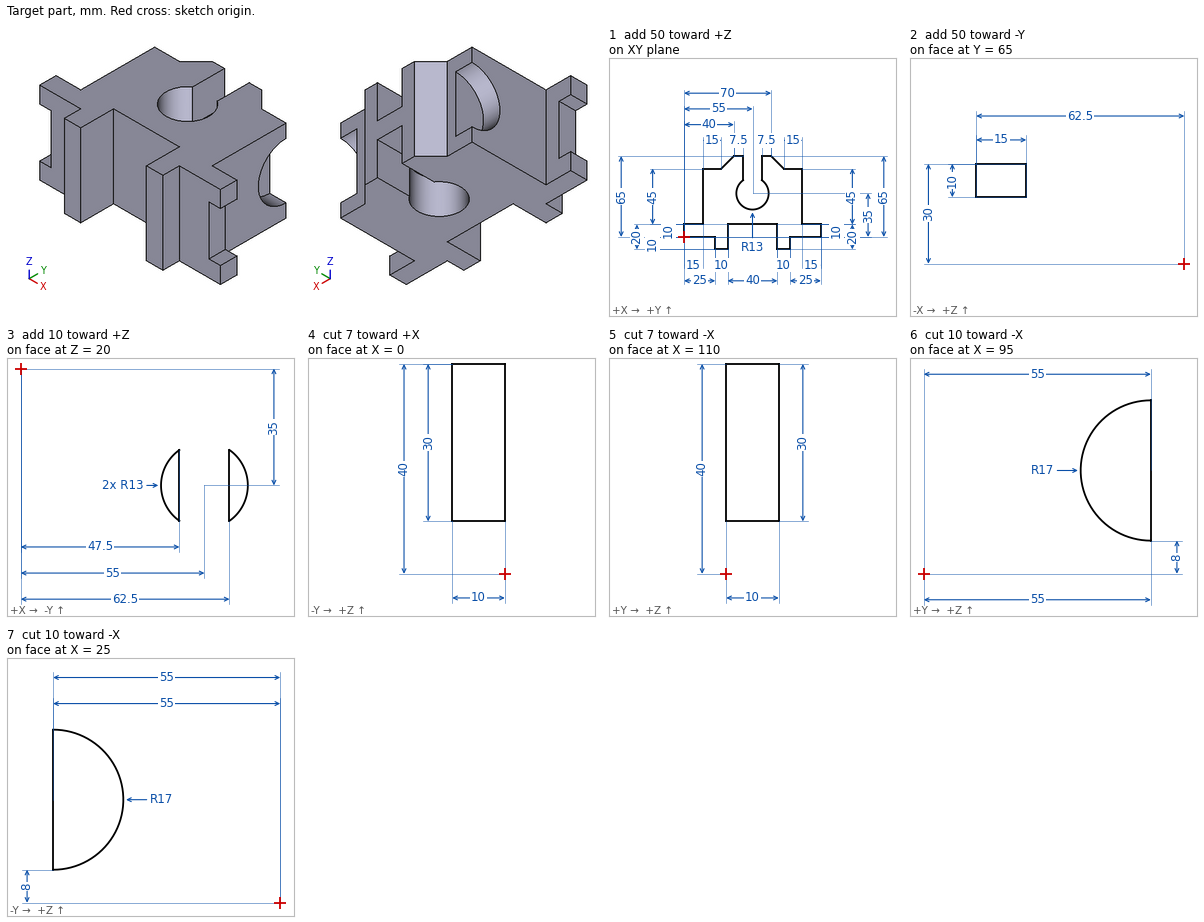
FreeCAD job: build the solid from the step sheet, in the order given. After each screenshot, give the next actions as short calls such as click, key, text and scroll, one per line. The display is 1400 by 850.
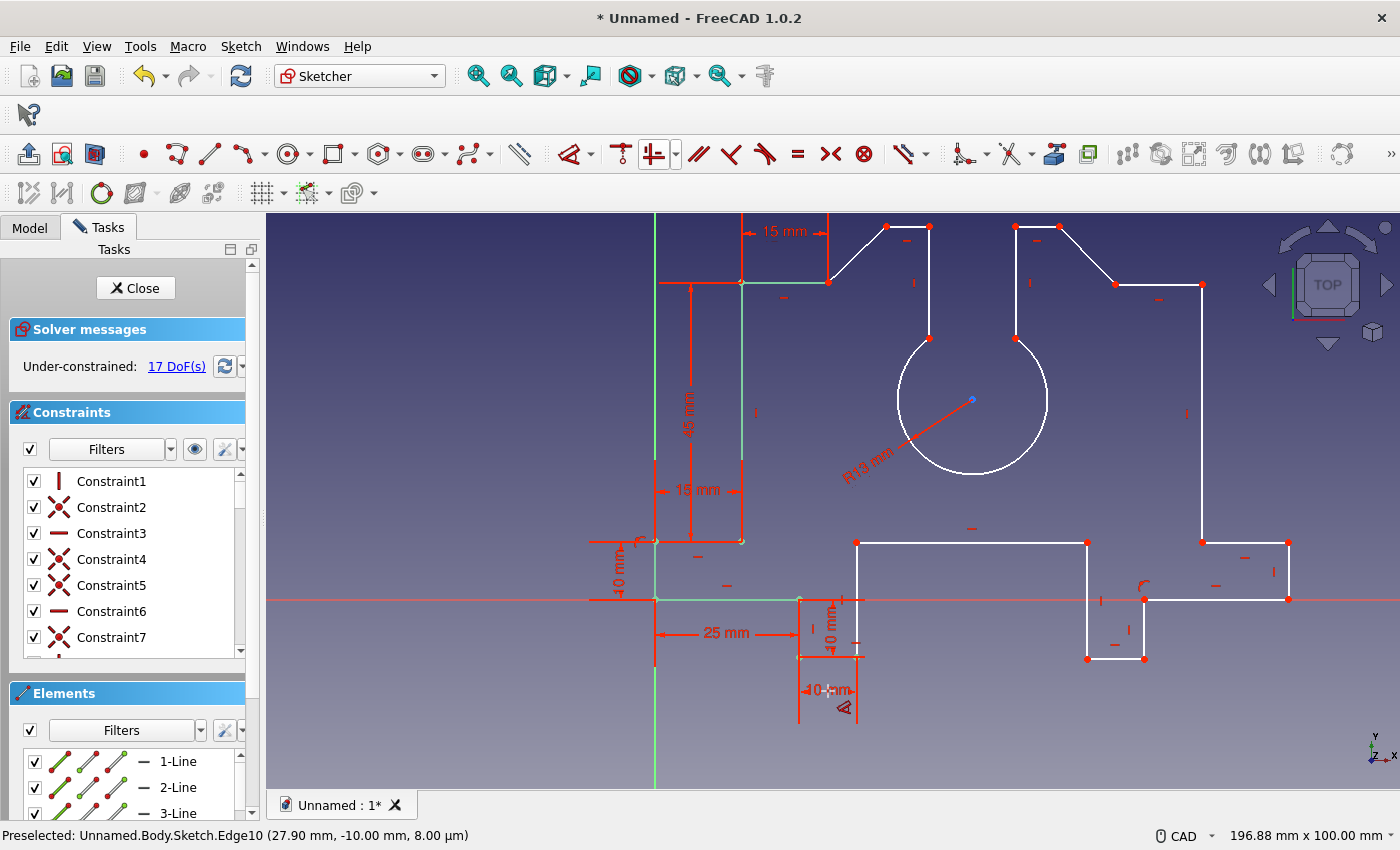
click(857, 623)
click(823, 574)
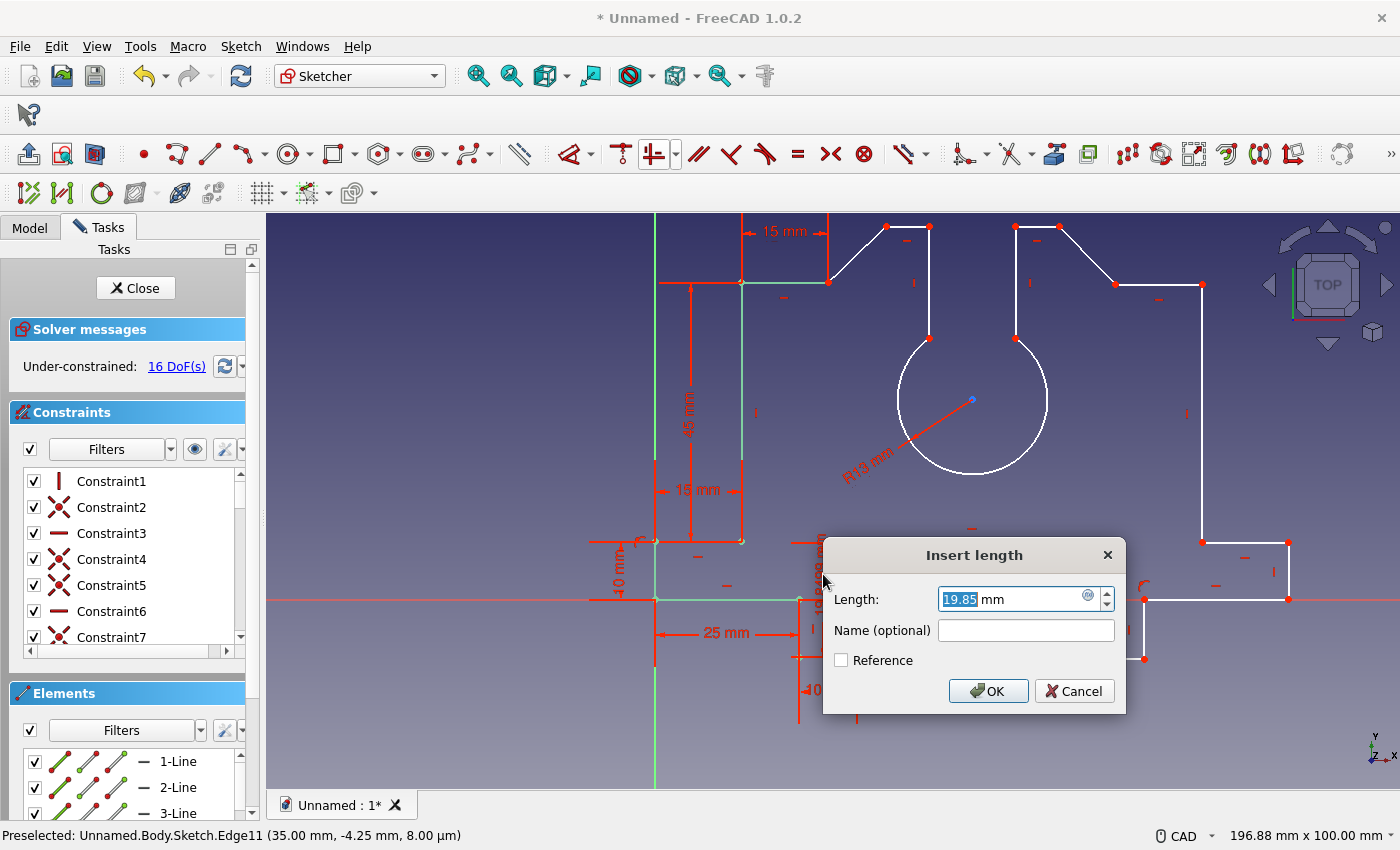
text(20)
key(Return)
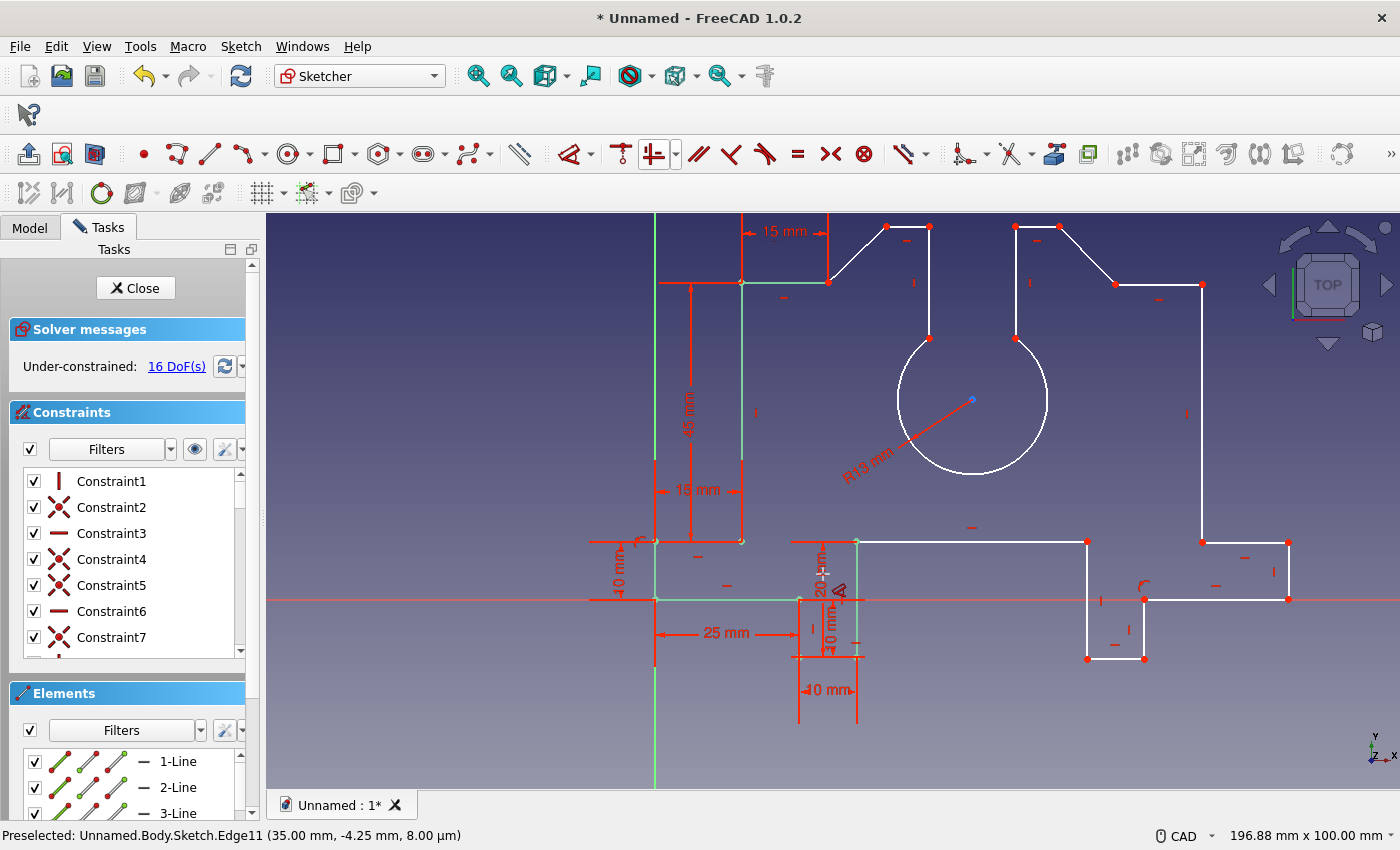
click(926, 542)
click(972, 576)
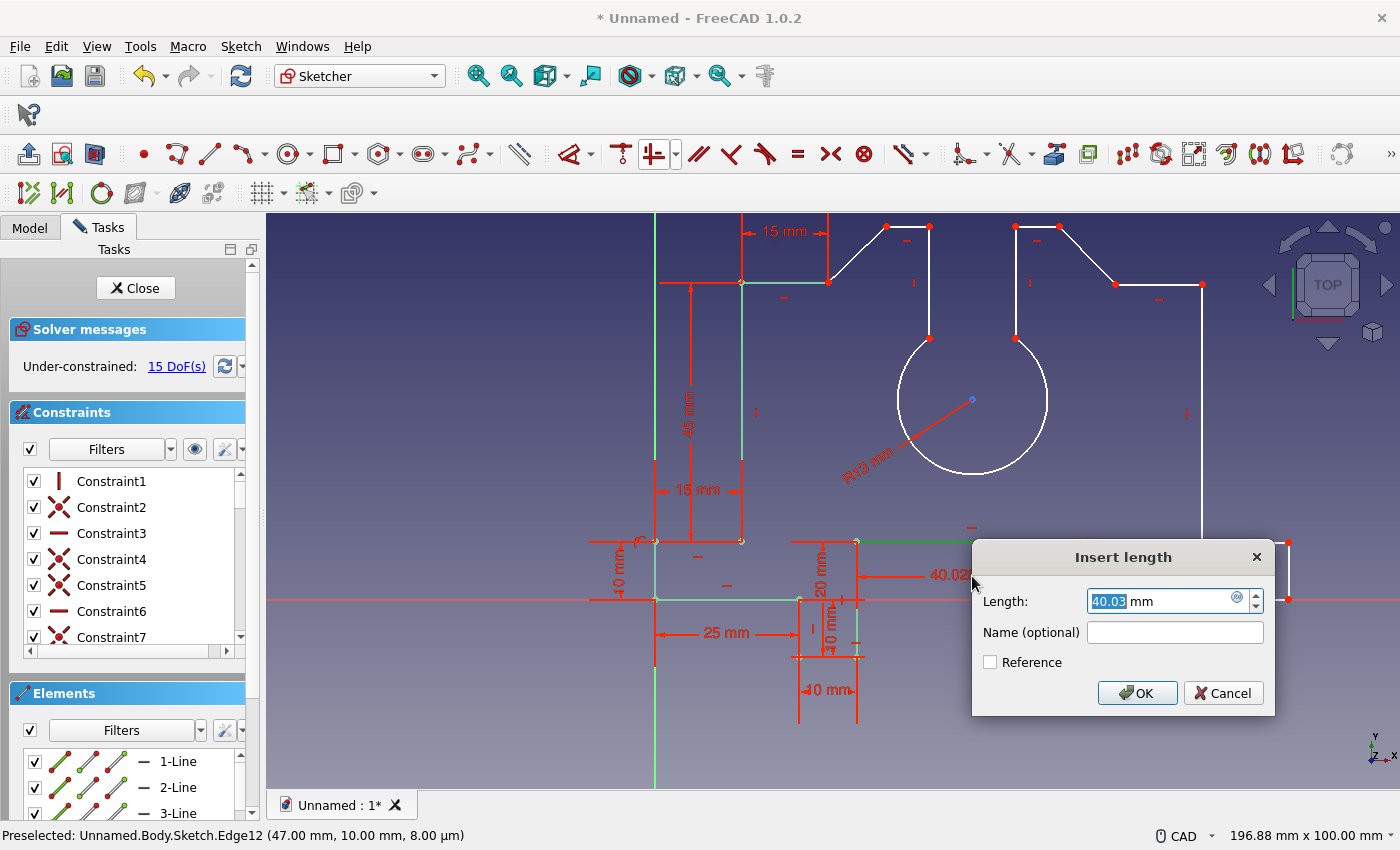
text(40)
key(Return)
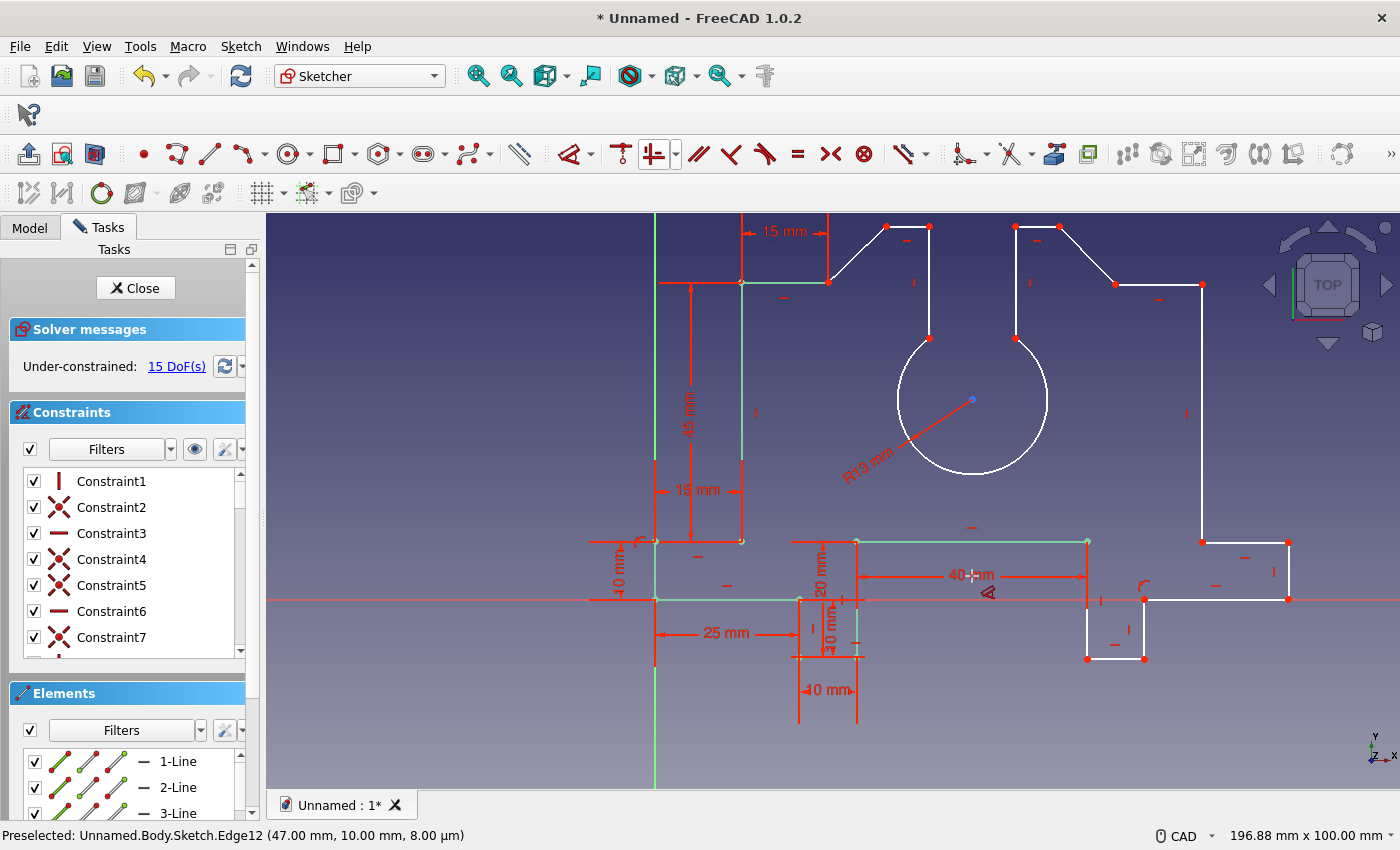
click(1087, 577)
click(1121, 574)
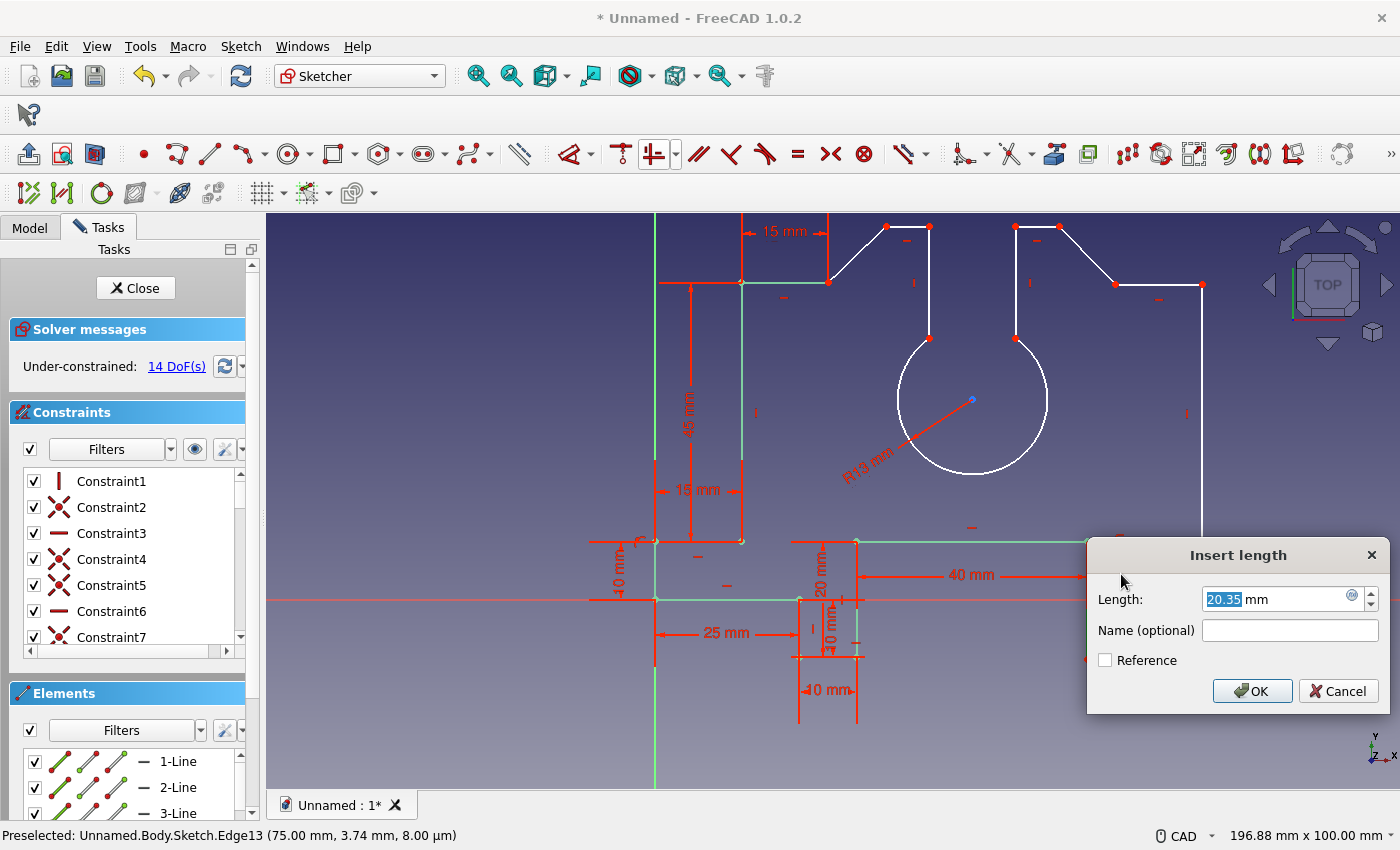
text(20)
key(Return)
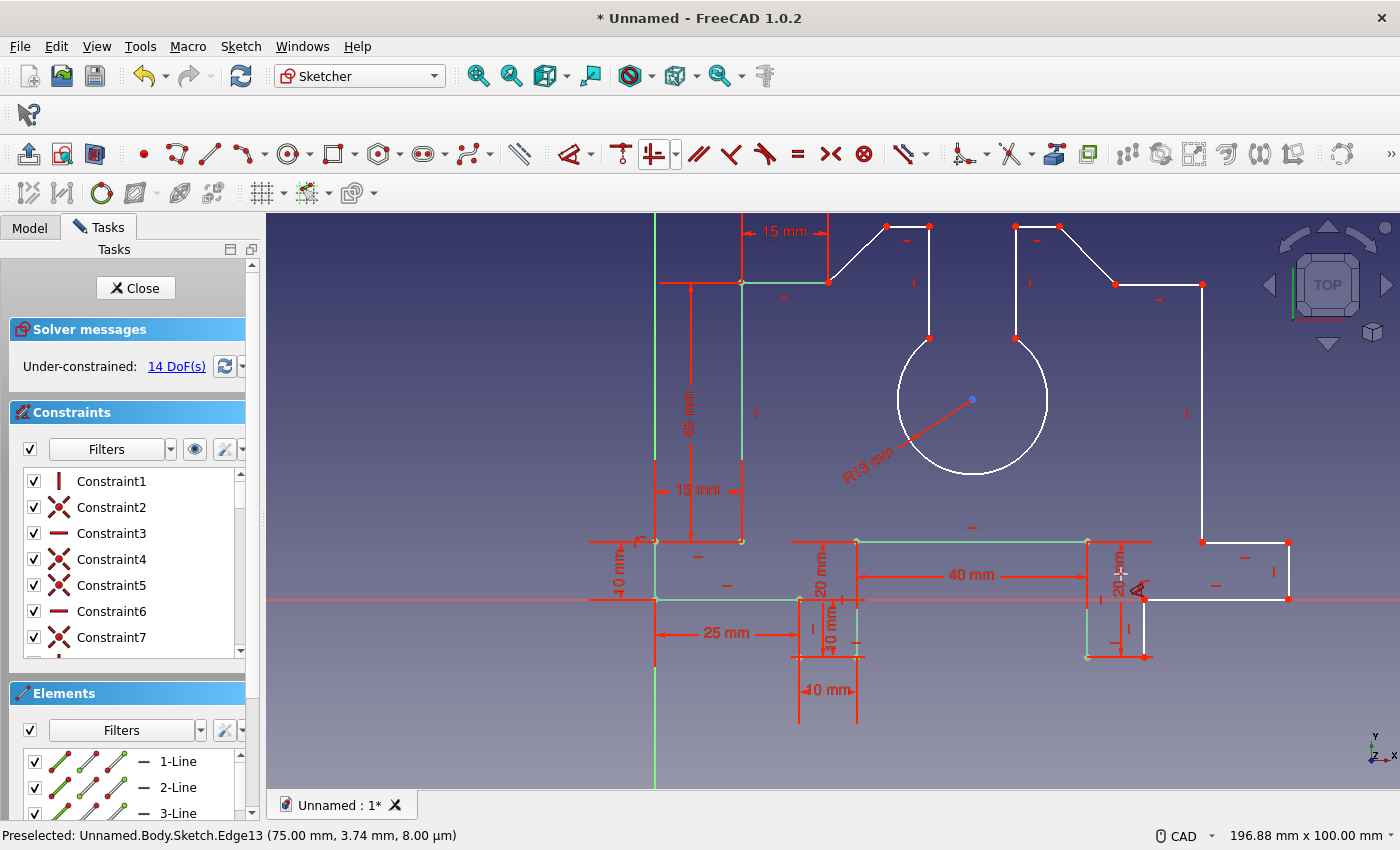
click(1104, 657)
click(1116, 691)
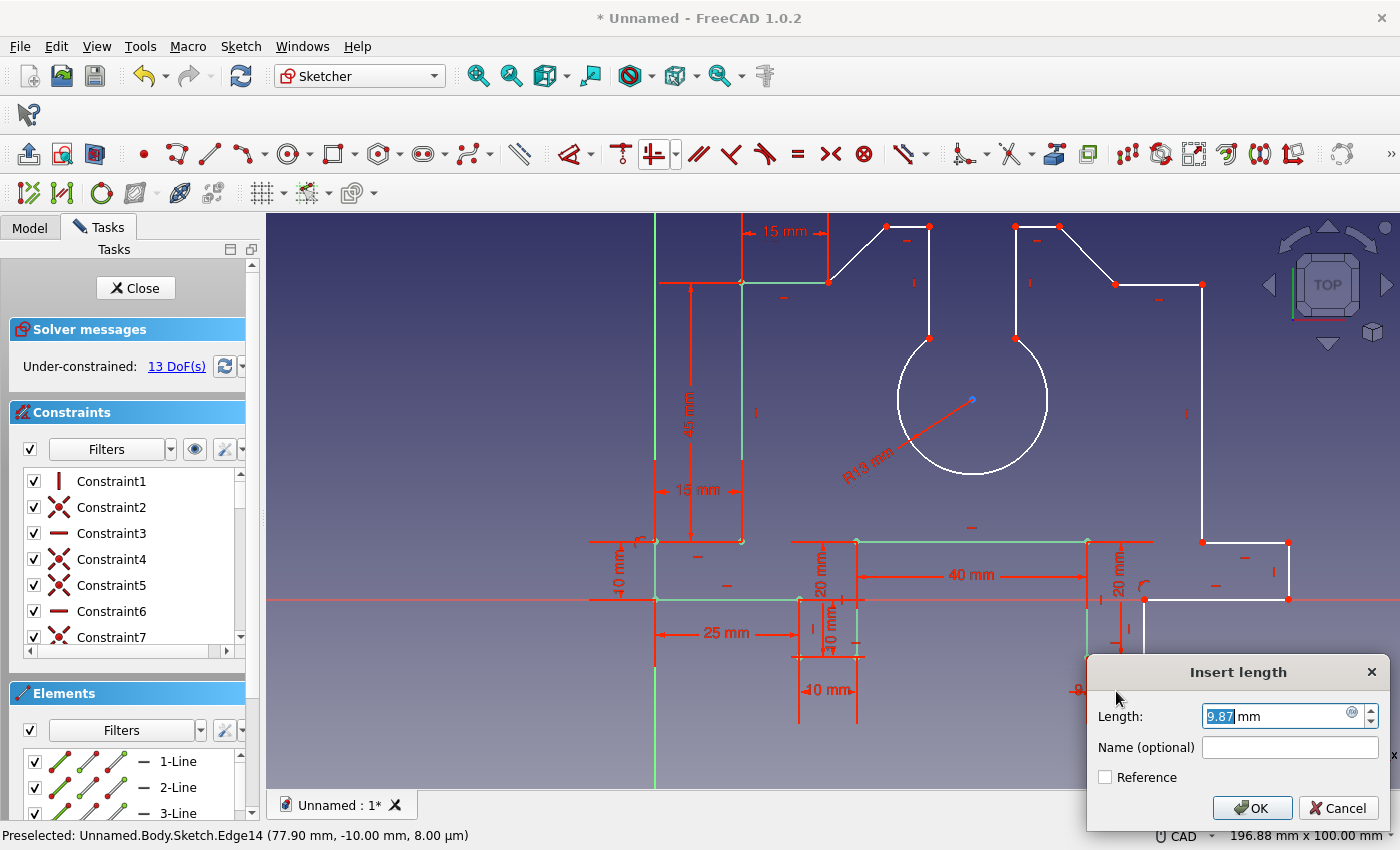
text(10)
key(Return)